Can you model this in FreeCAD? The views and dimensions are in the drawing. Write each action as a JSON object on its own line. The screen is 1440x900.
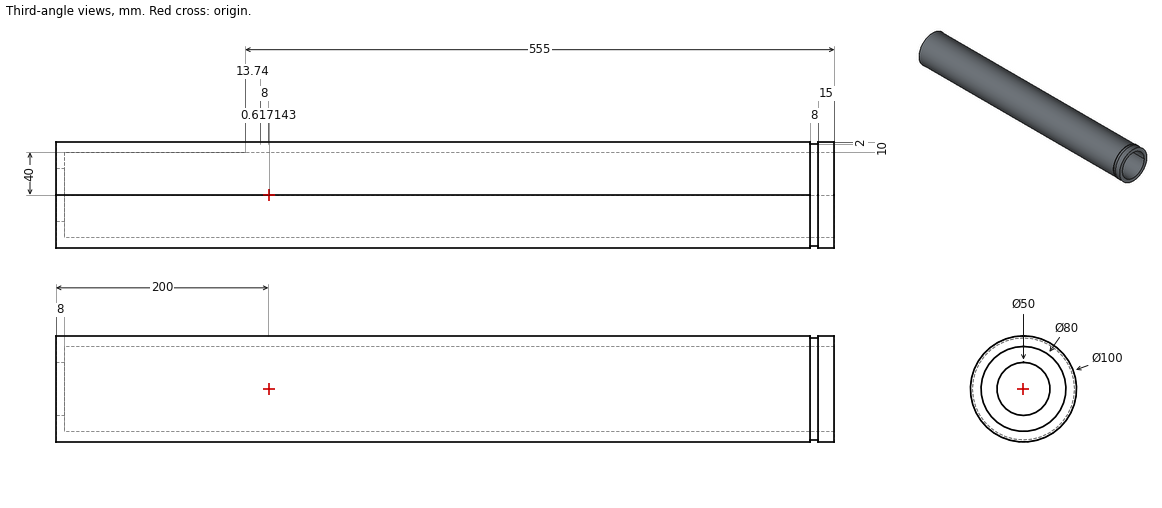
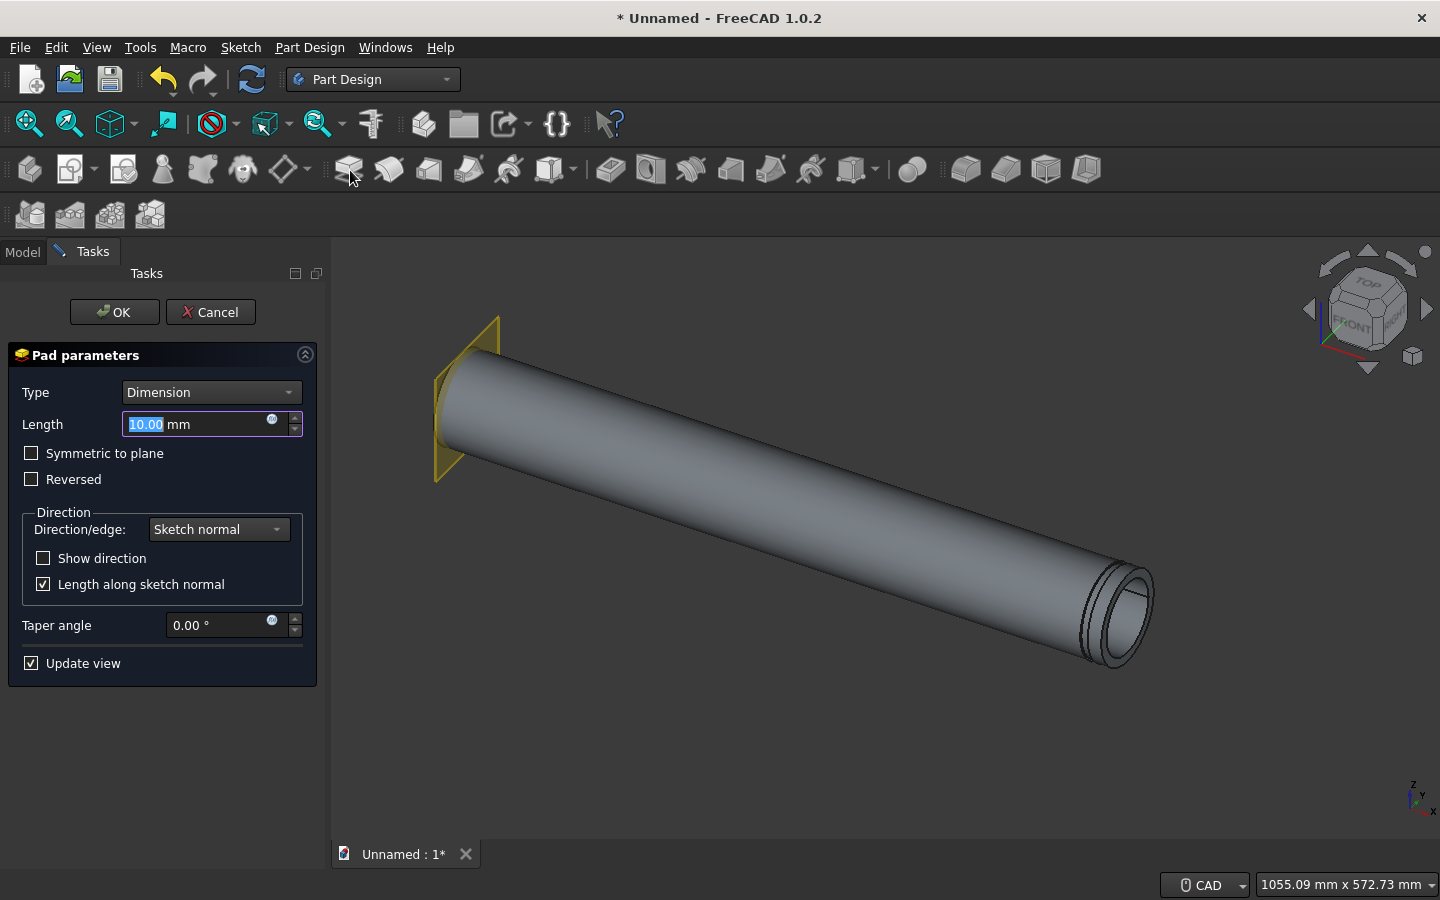
{"action": "type", "text": "8"}
{"action": "key", "text": "Tab"}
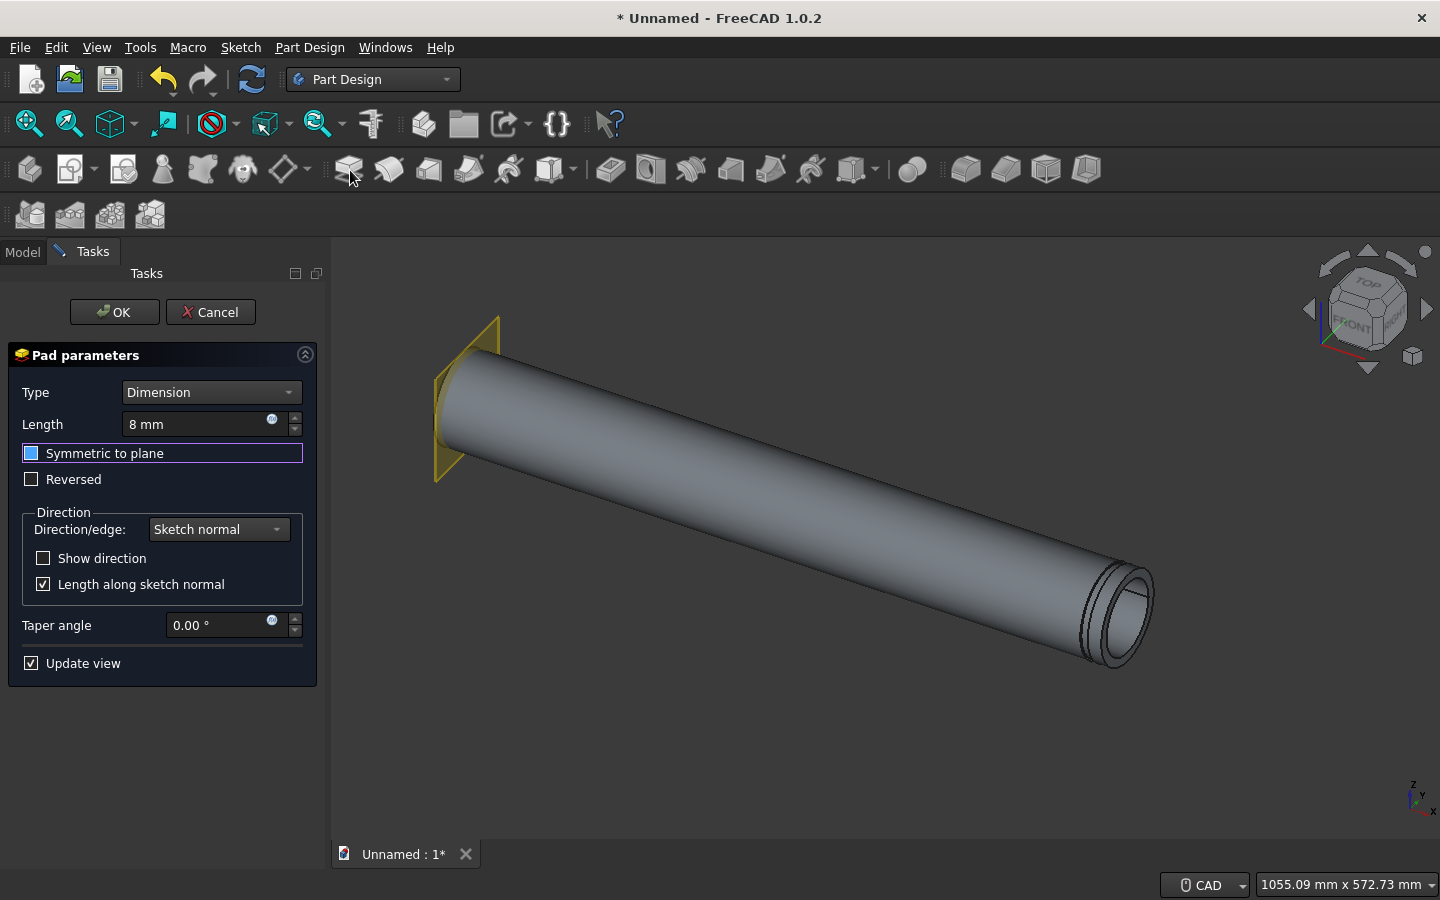
{"action": "left_click", "coordinate": [30, 479]}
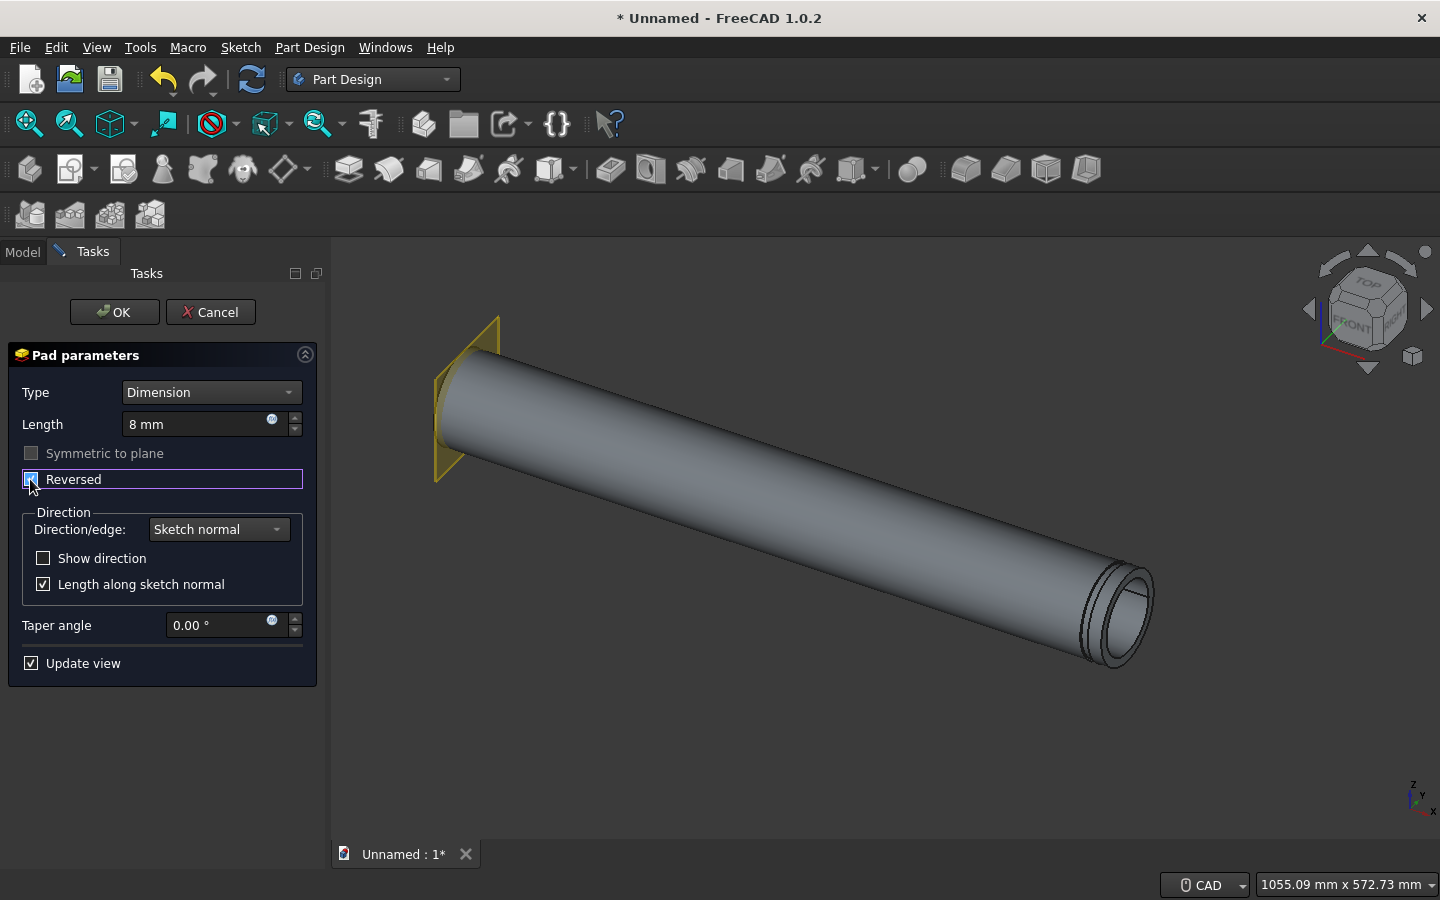
{"action": "left_click", "coordinate": [115, 312]}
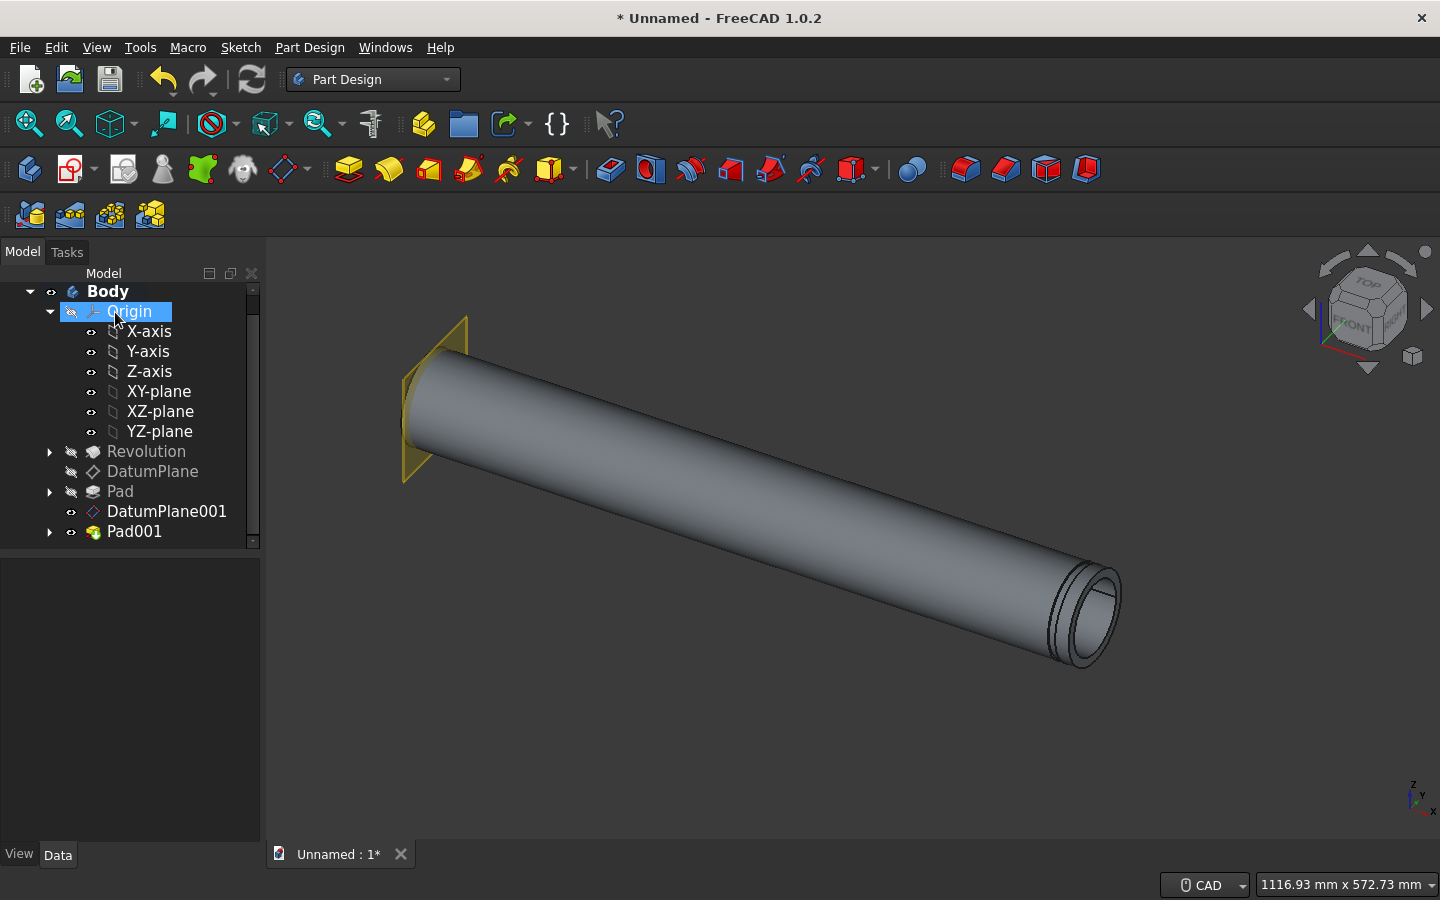
{"action": "left_click", "coordinate": [116, 512]}
{"action": "key", "text": "space"}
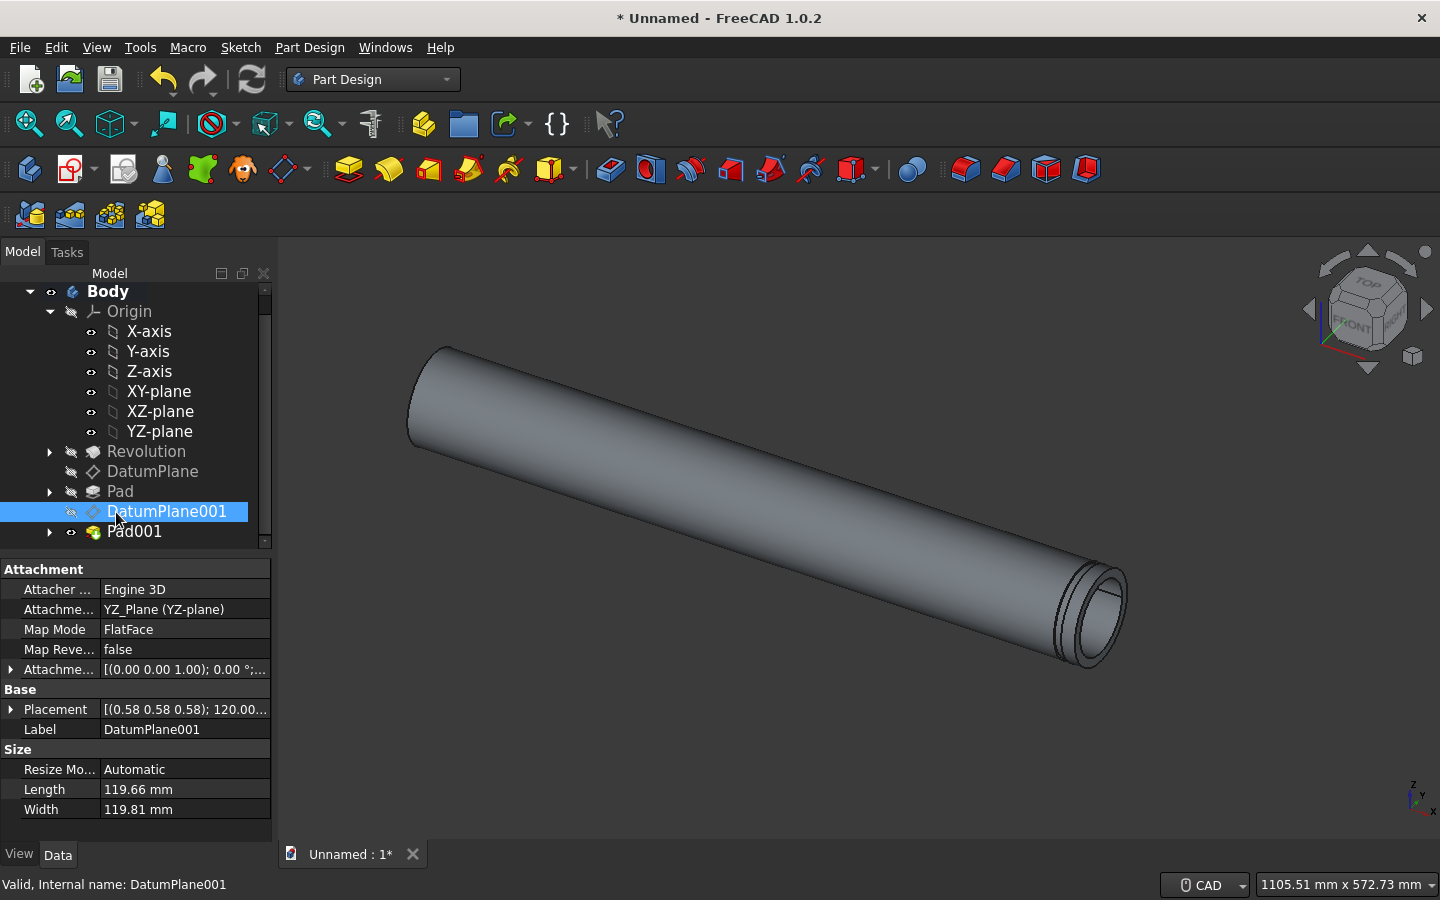
{"action": "key", "text": "0"}